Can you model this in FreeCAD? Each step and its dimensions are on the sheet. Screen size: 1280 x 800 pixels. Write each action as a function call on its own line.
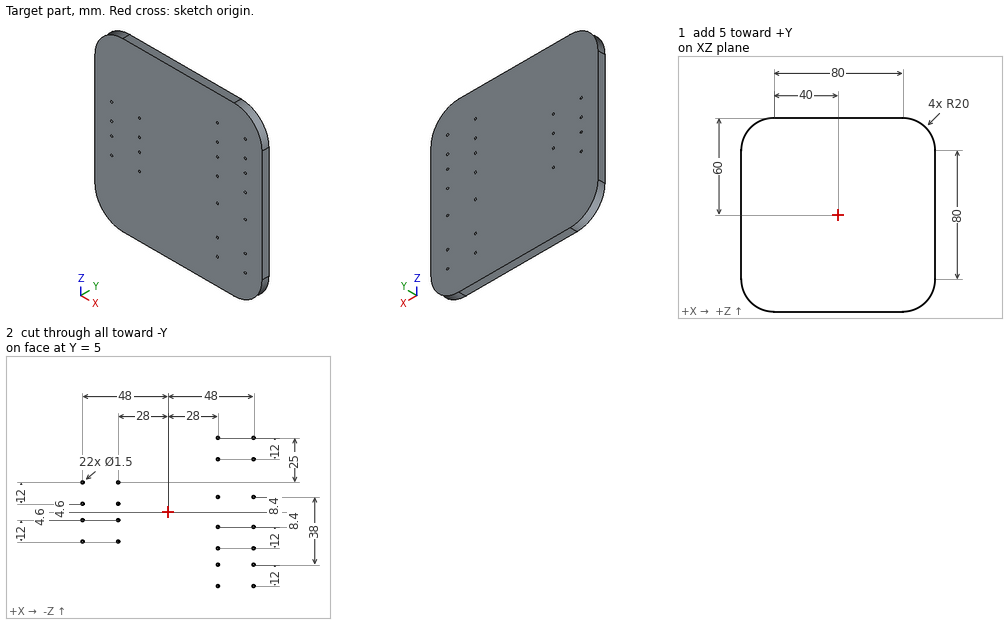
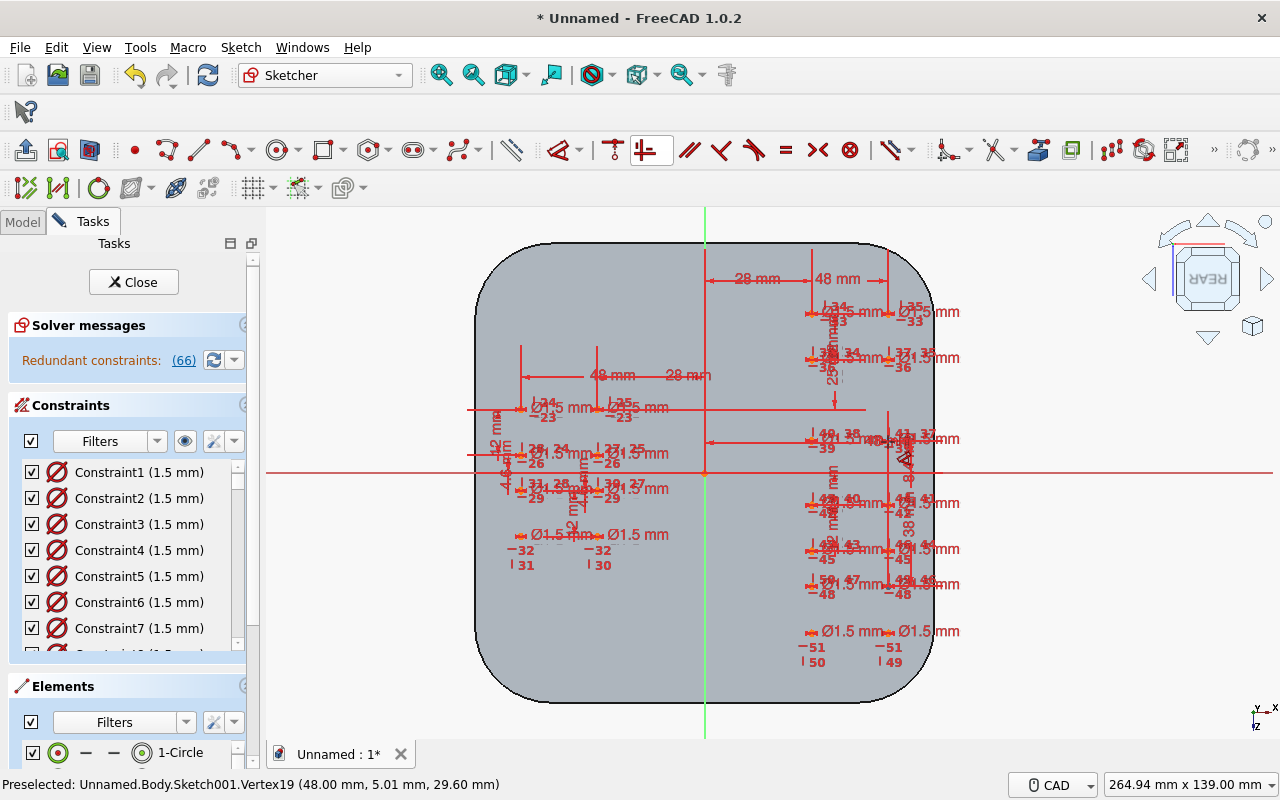
click(888, 633)
click(922, 610)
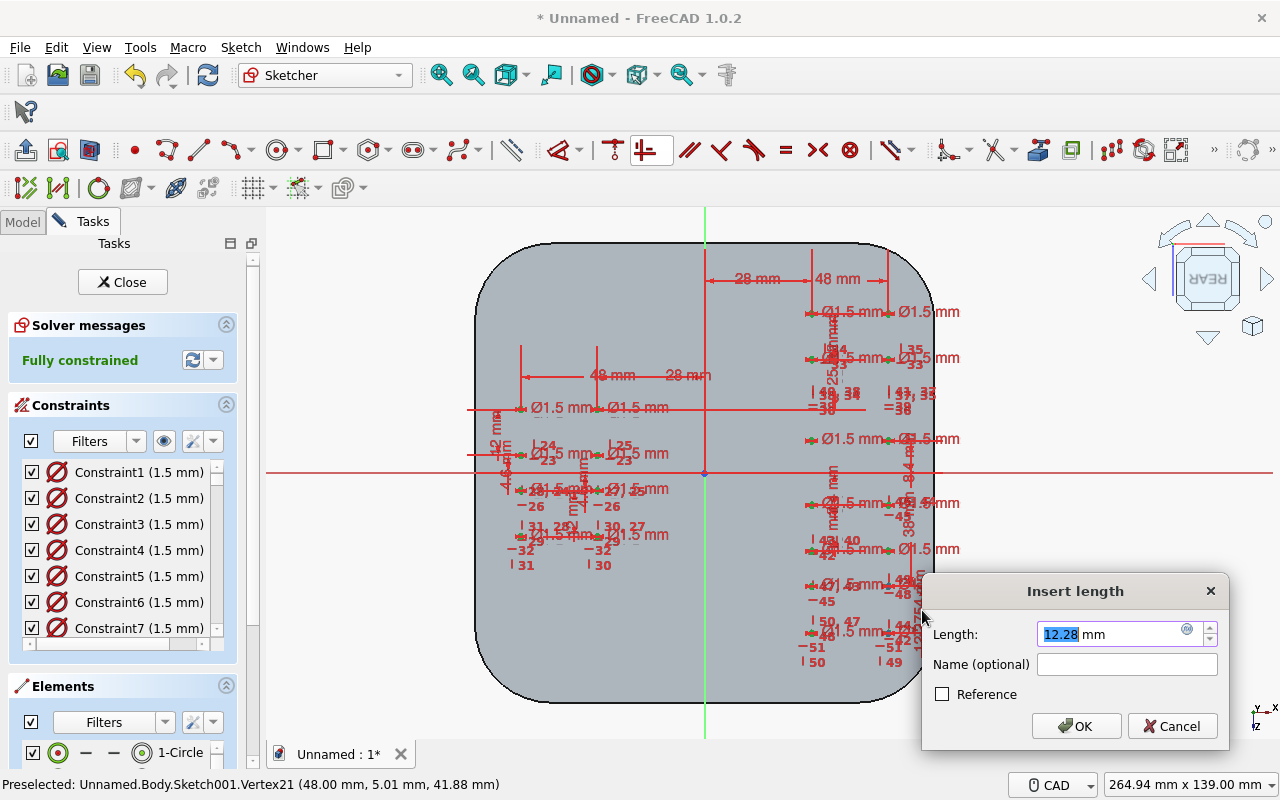
text(12)
key(Return)
key(Escape)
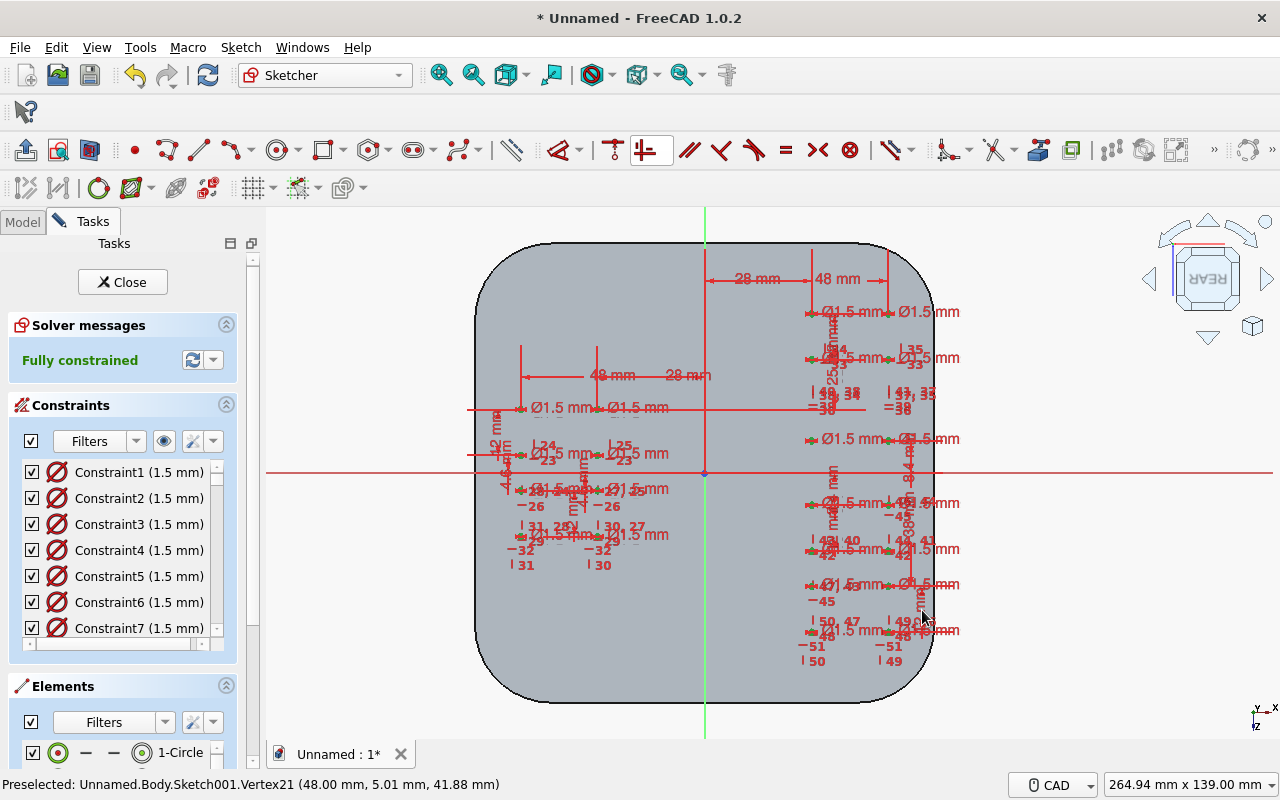
click(123, 282)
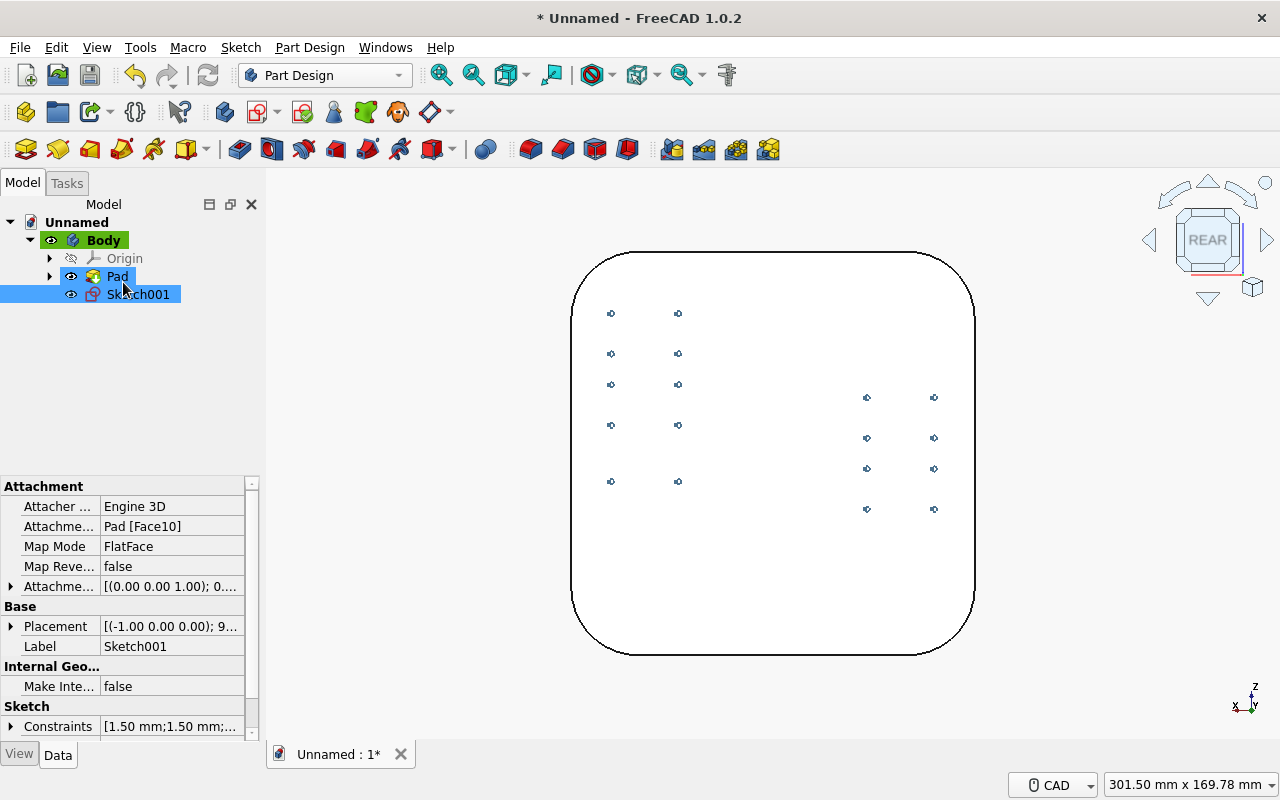
click(240, 150)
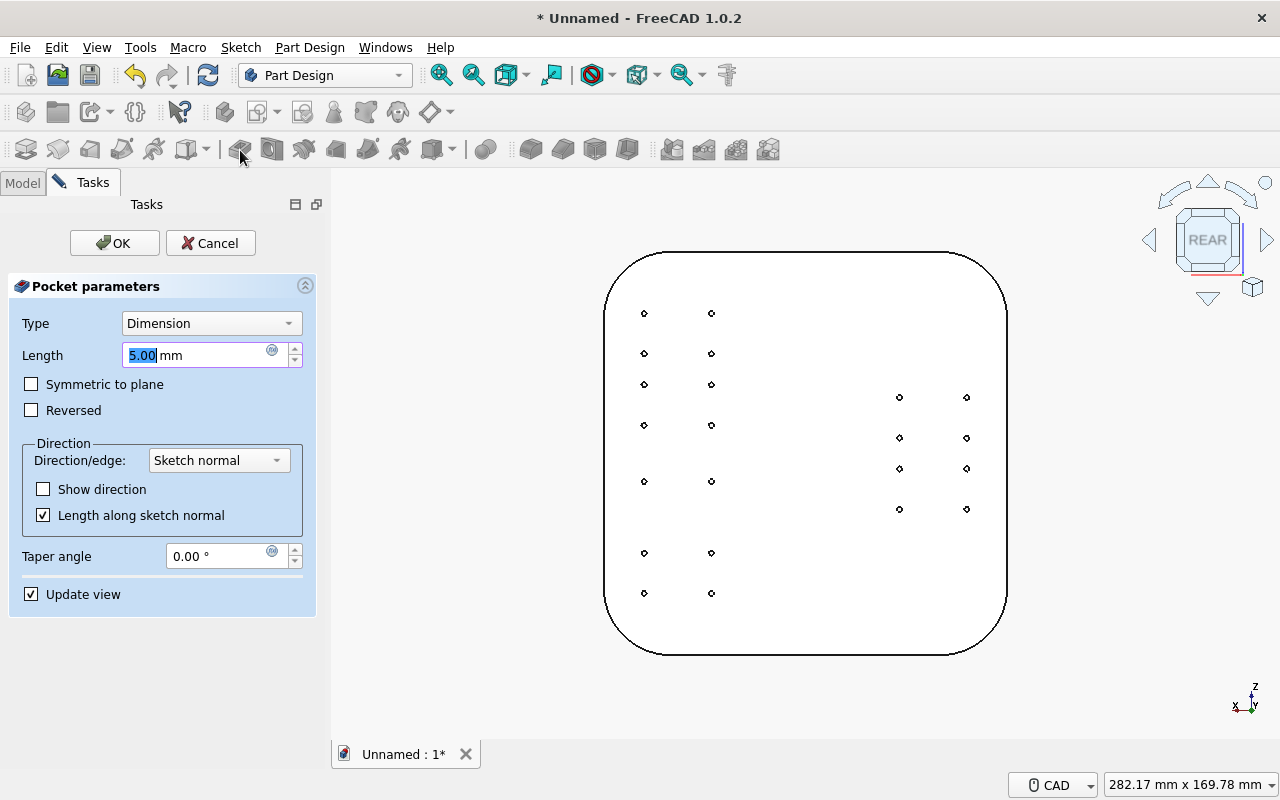
click(212, 324)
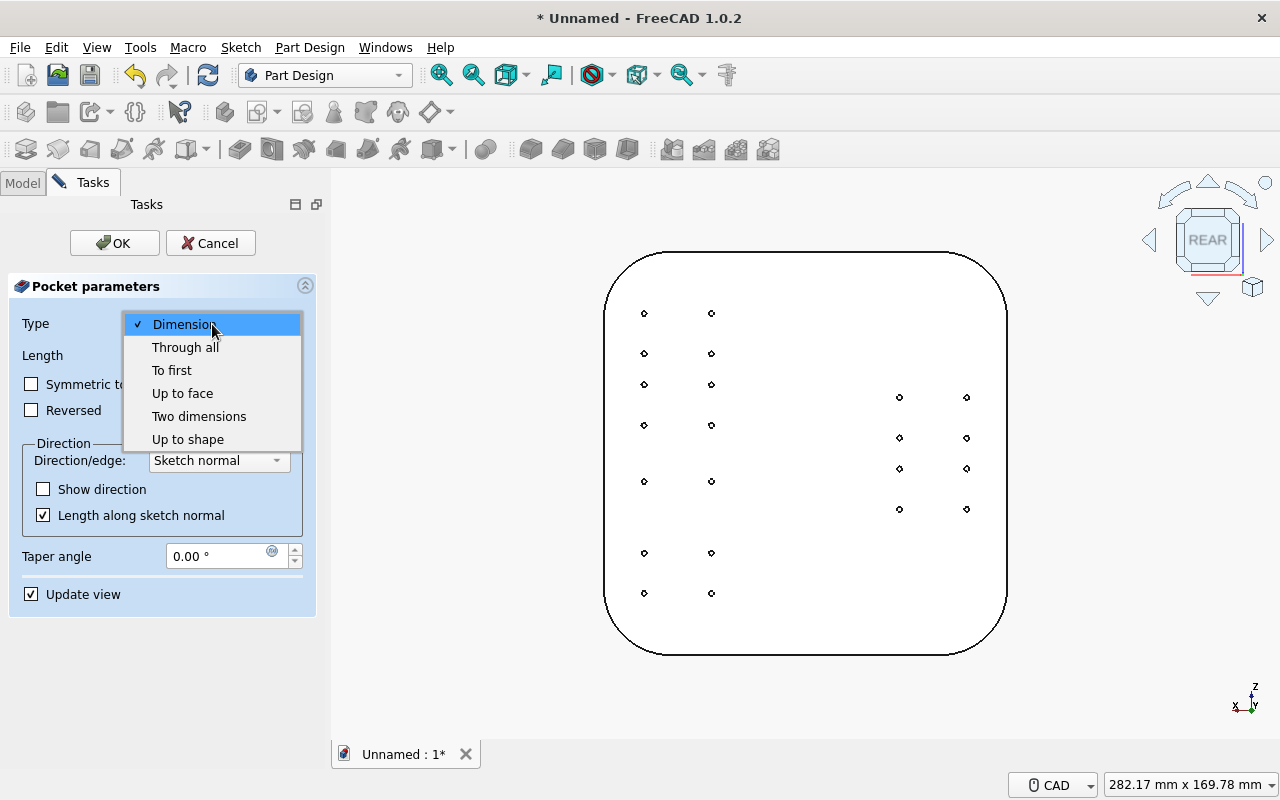
click(212, 348)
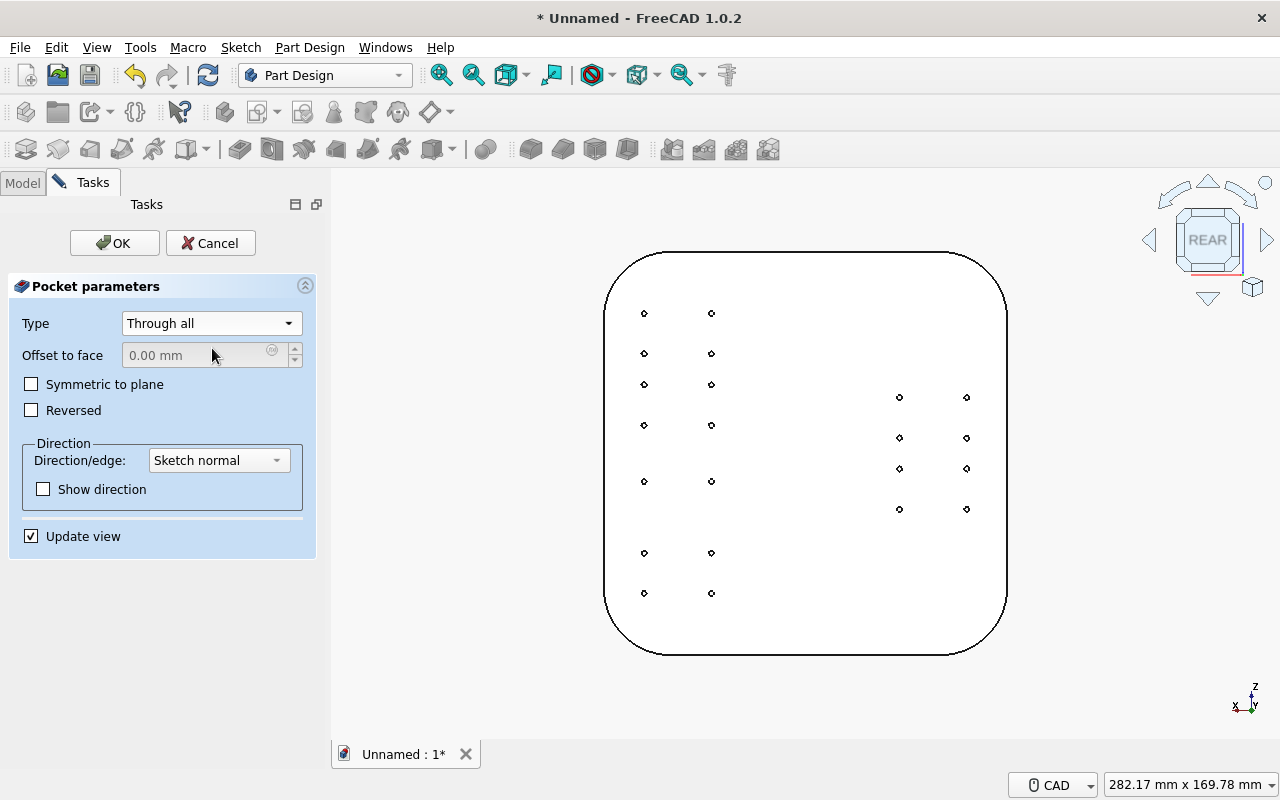
click(115, 243)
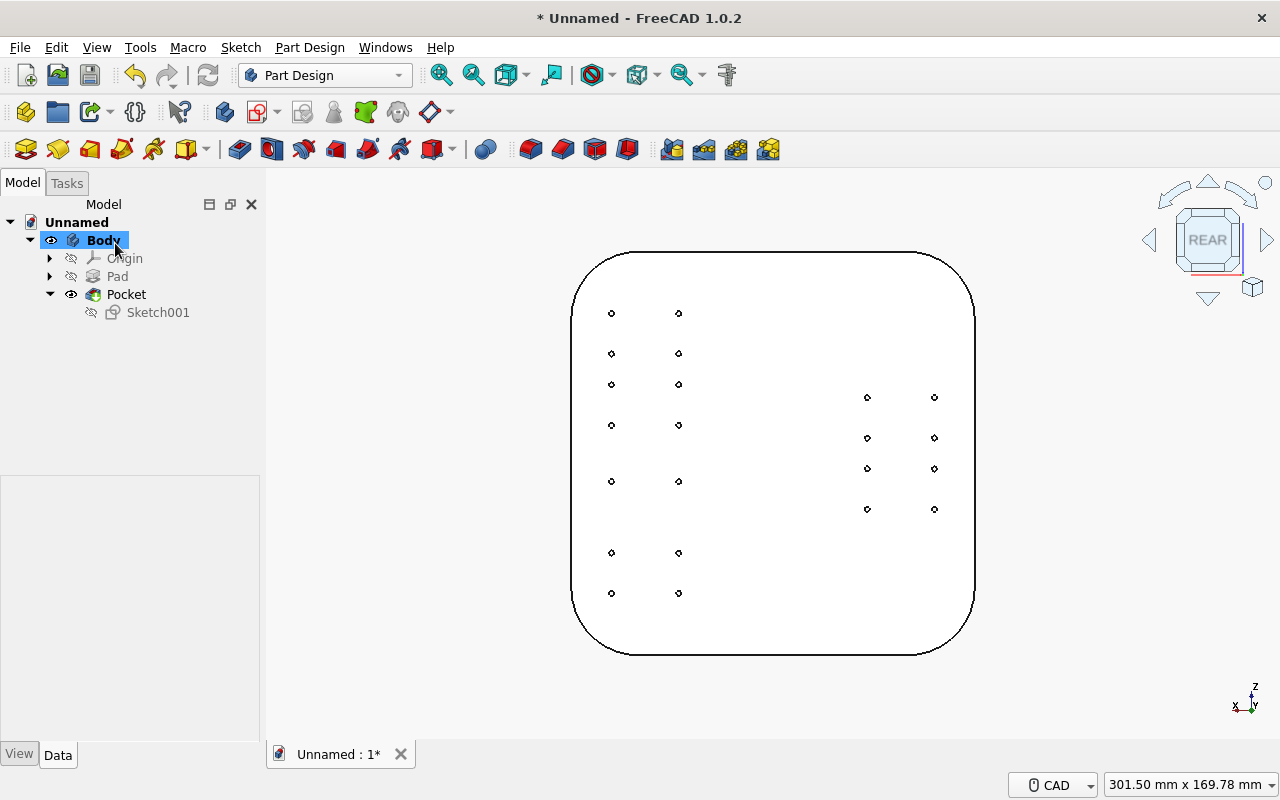
key(0)